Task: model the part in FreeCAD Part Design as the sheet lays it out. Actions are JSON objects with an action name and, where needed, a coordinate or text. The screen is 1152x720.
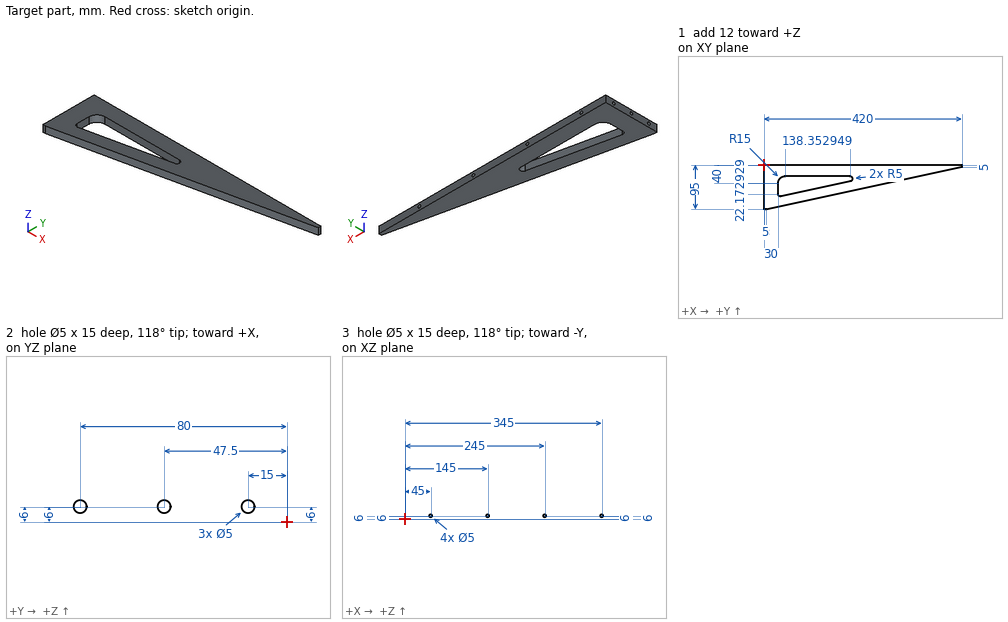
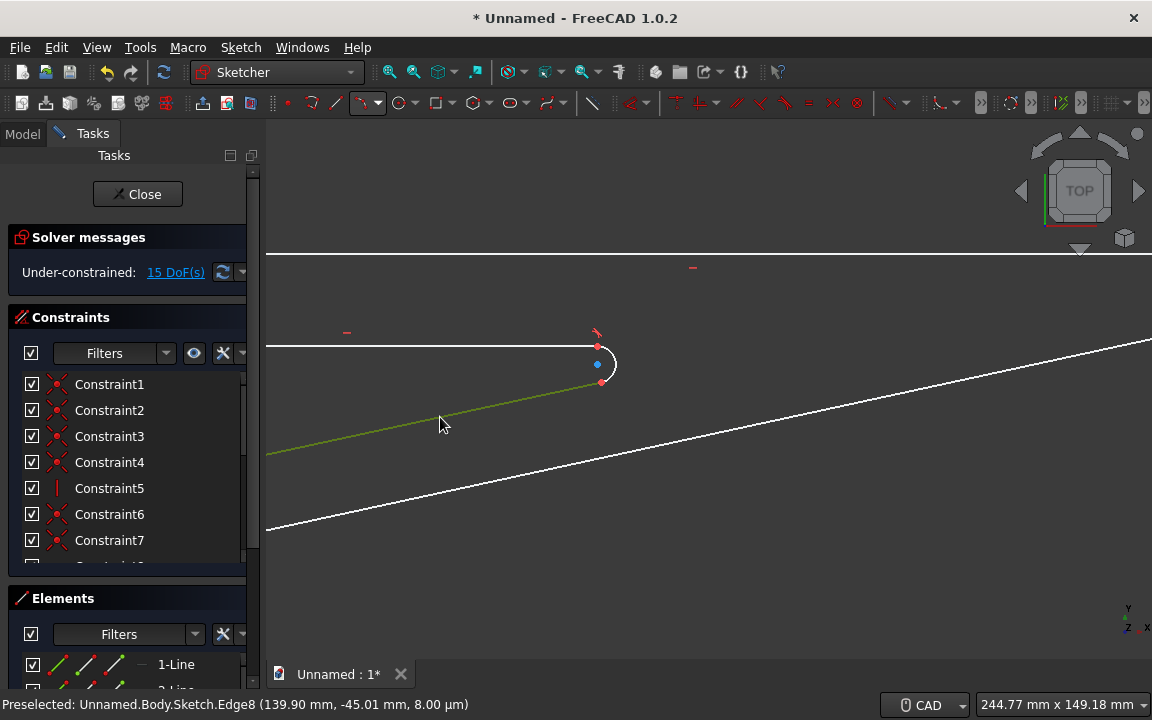
{"action": "left_click", "coordinate": [614, 373]}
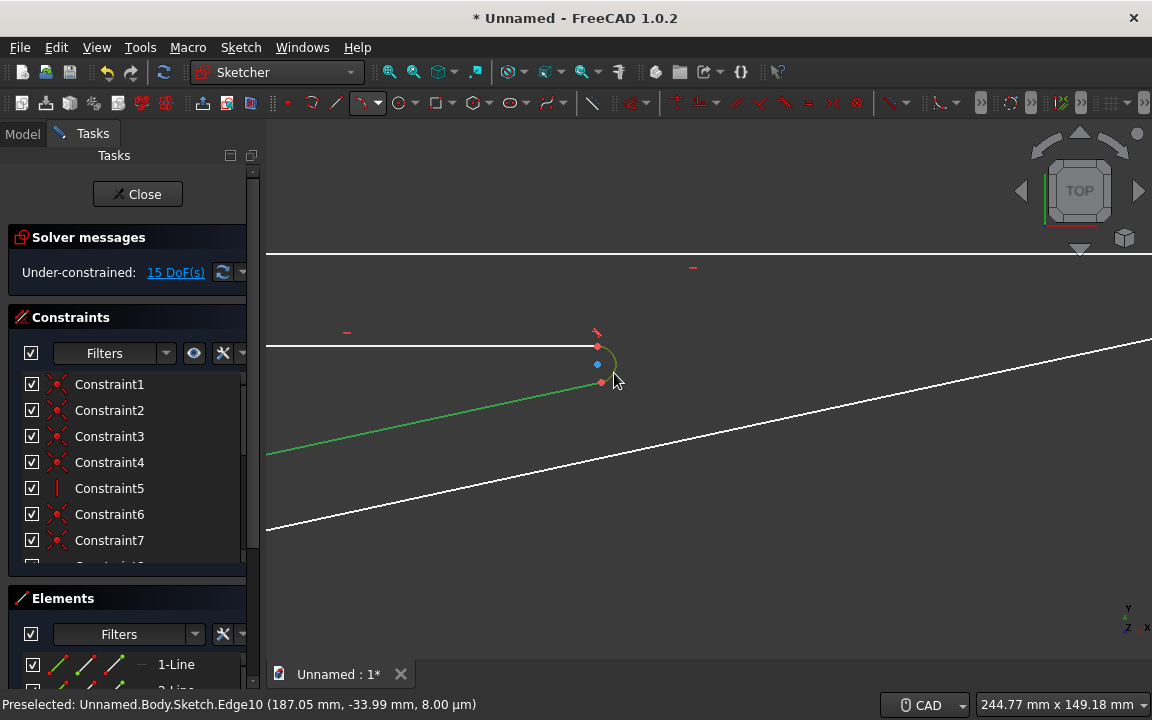
{"action": "left_click", "coordinate": [786, 104]}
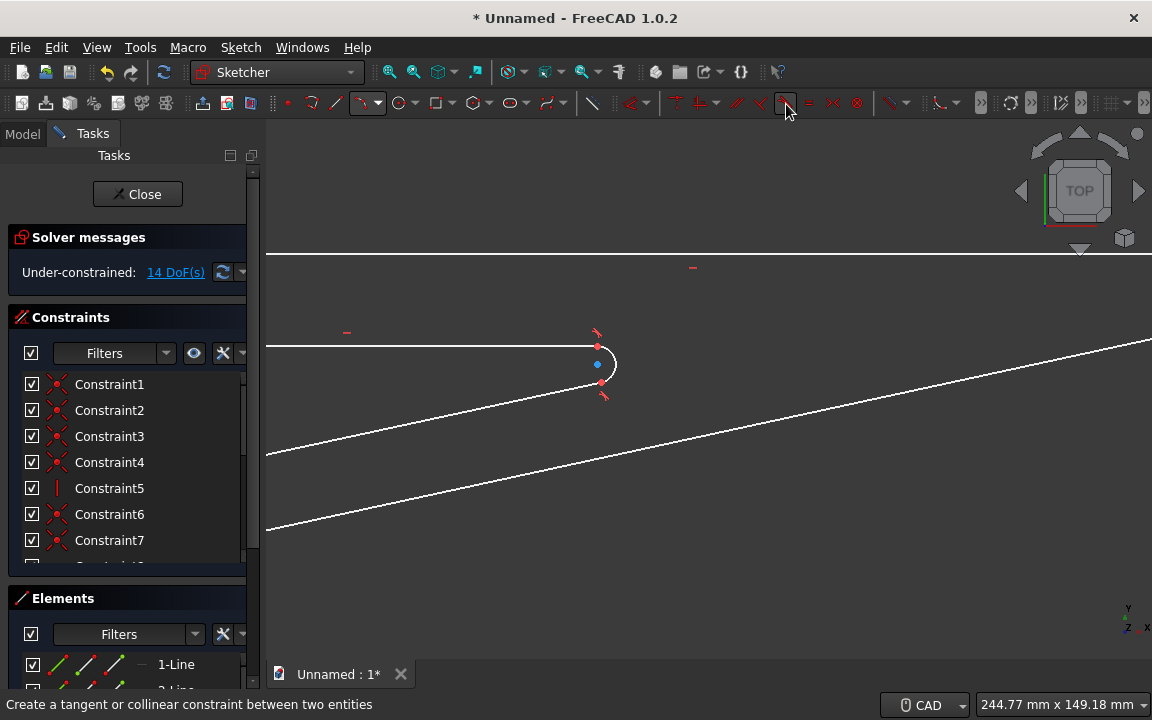
{"action": "left_click", "coordinate": [440, 417]}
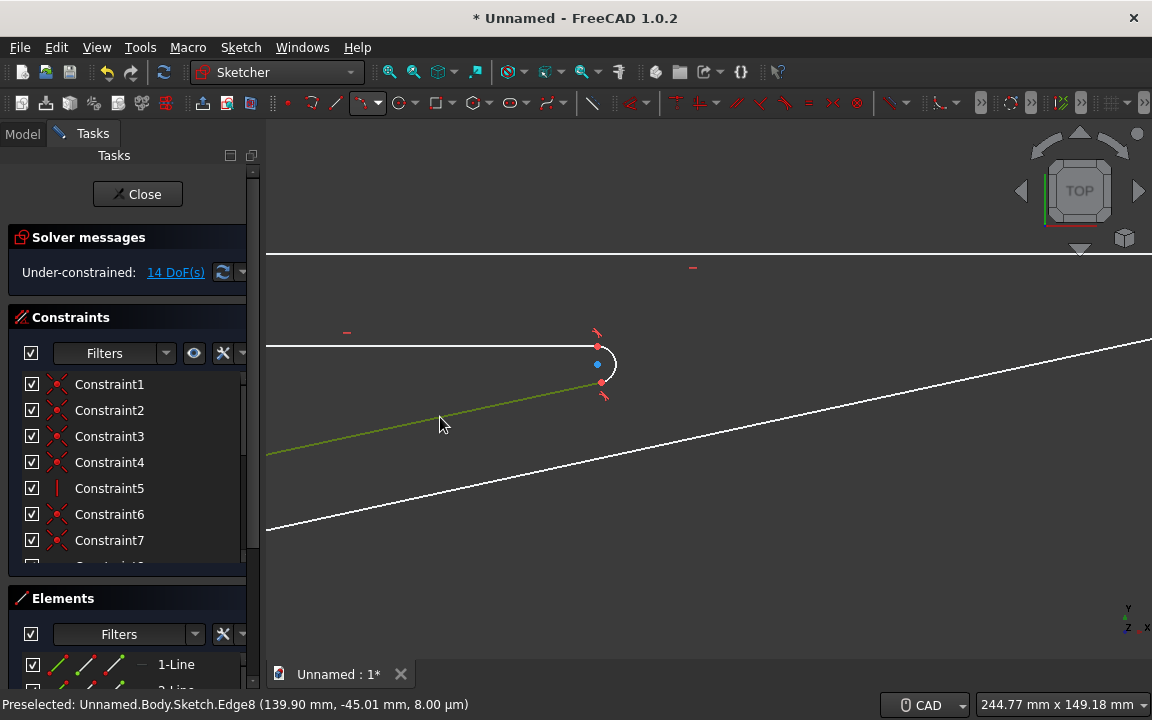
{"action": "scroll", "coordinate": [618, 373], "scroll_direction": "down", "scroll_amount": 6}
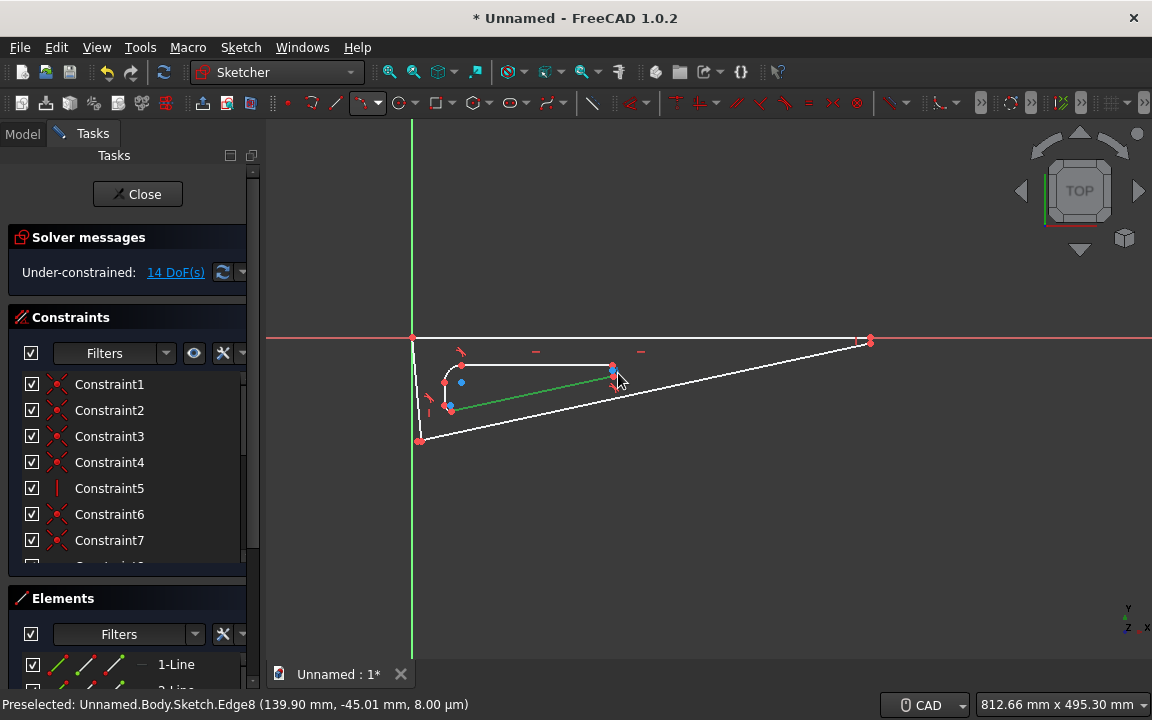
{"action": "scroll", "coordinate": [445, 408], "scroll_direction": "up", "scroll_amount": 8}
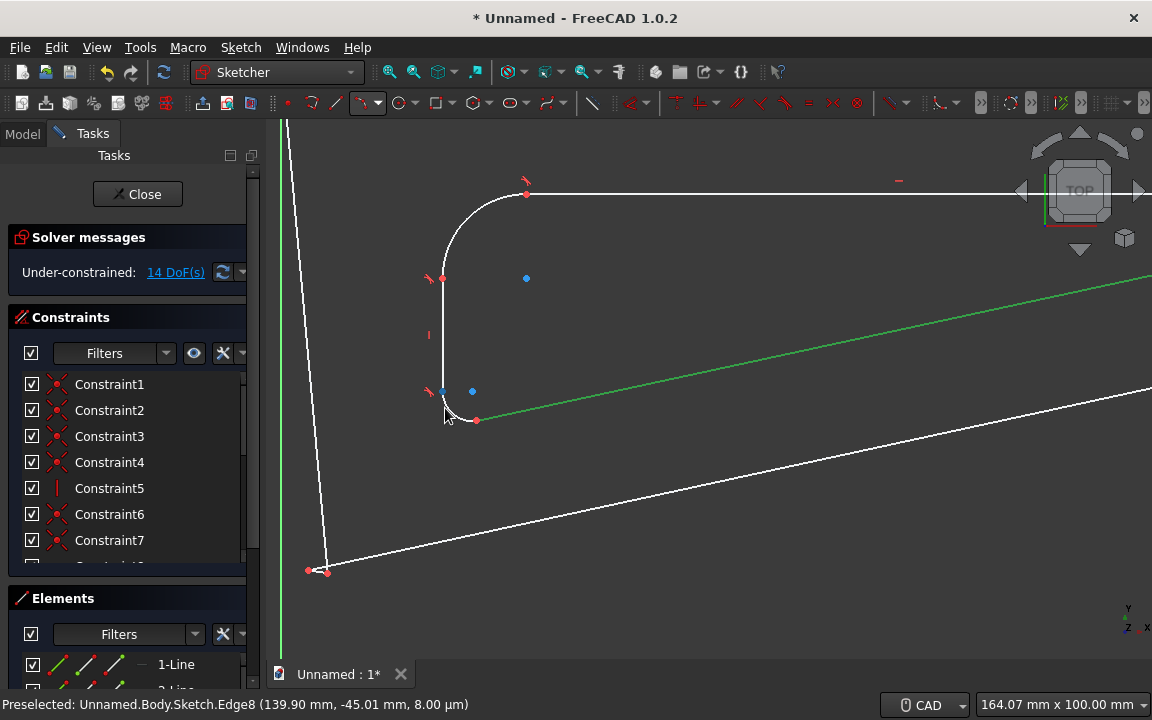
{"action": "left_click", "coordinate": [447, 406]}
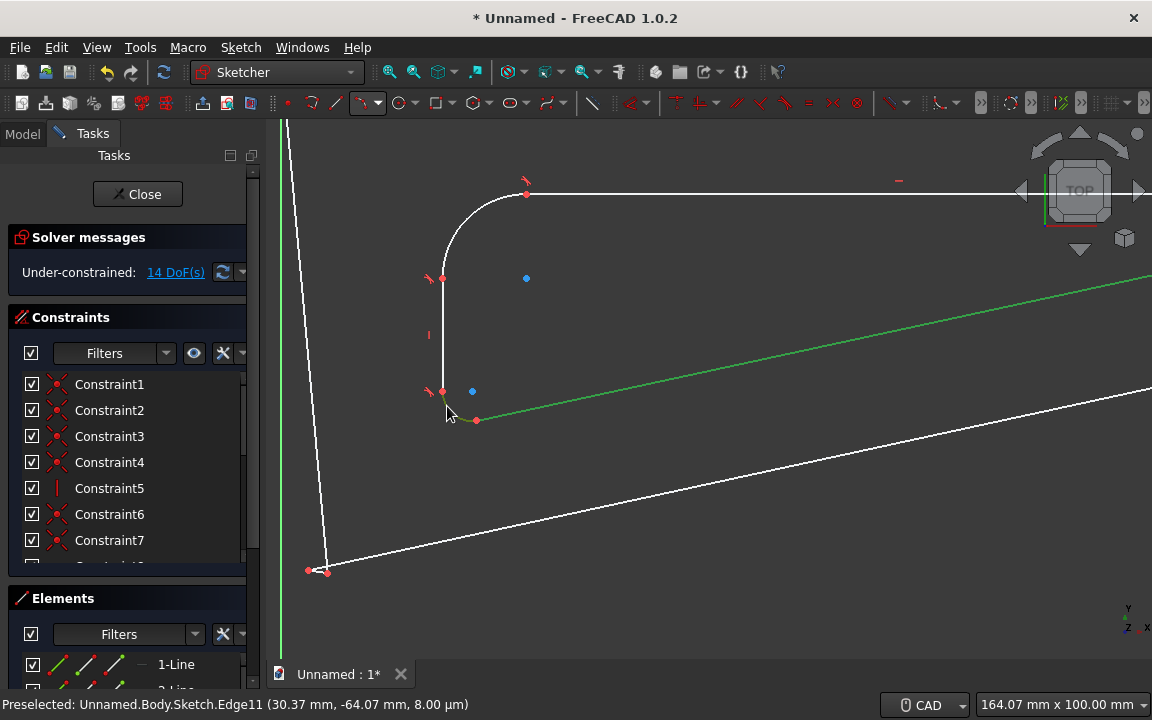
{"action": "left_click", "coordinate": [786, 104]}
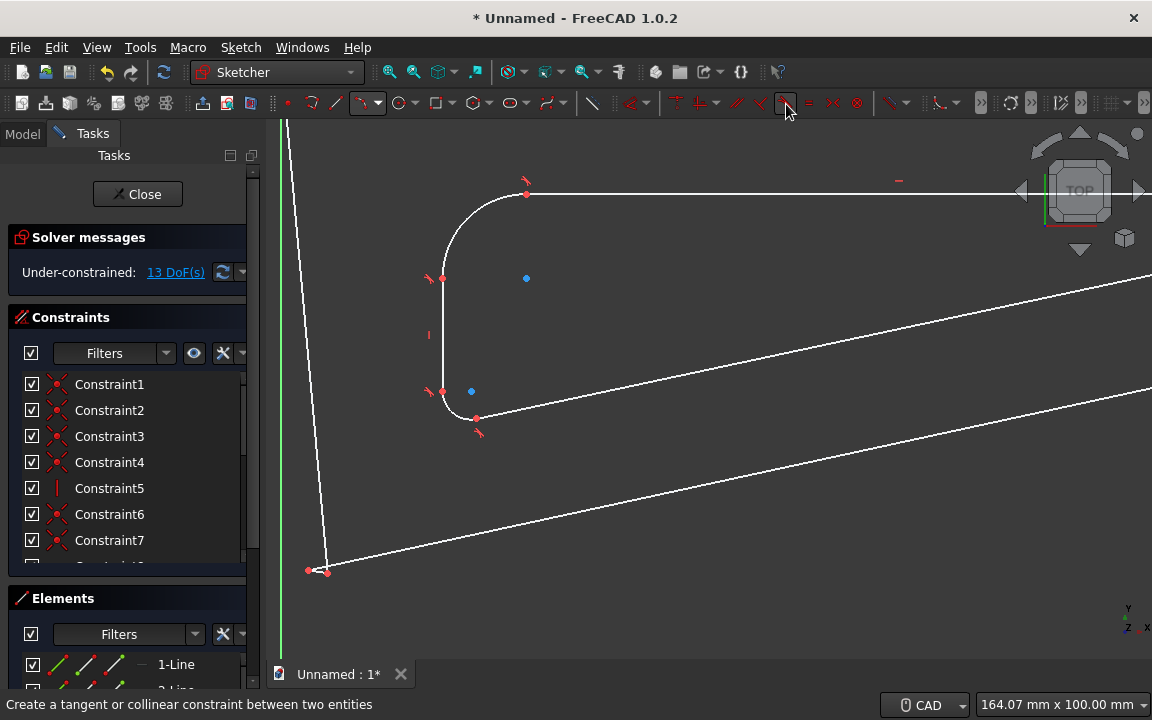
{"action": "left_click", "coordinate": [295, 212]}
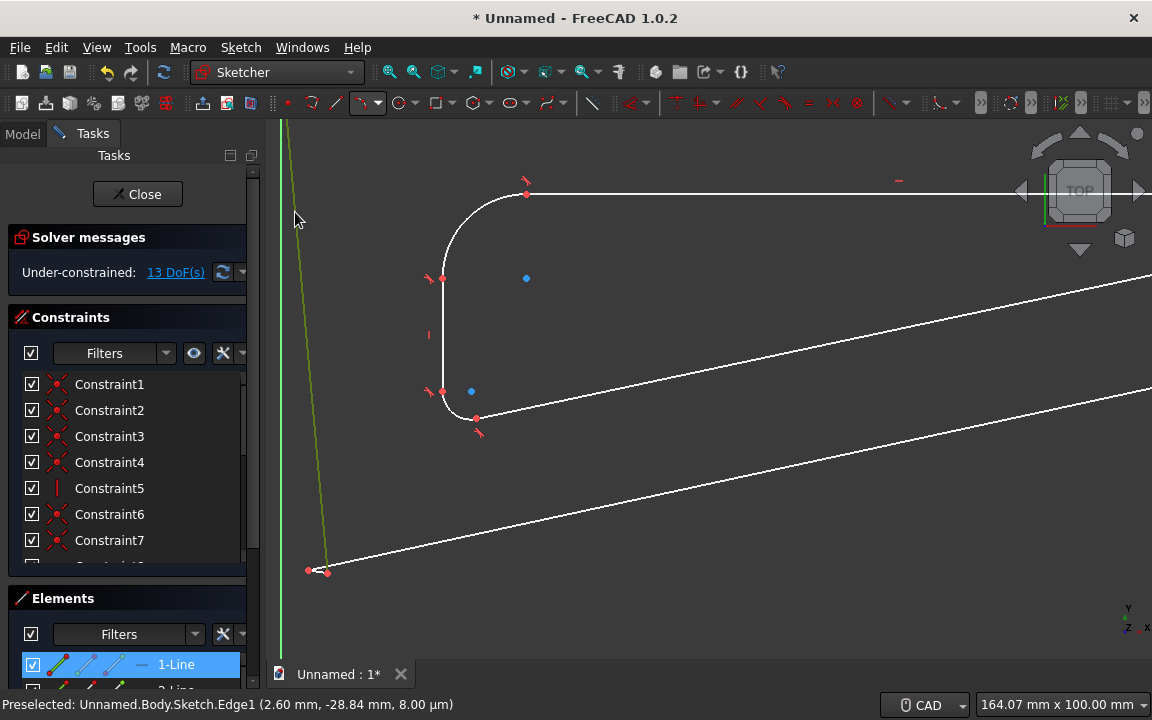
{"action": "key", "text": "v"}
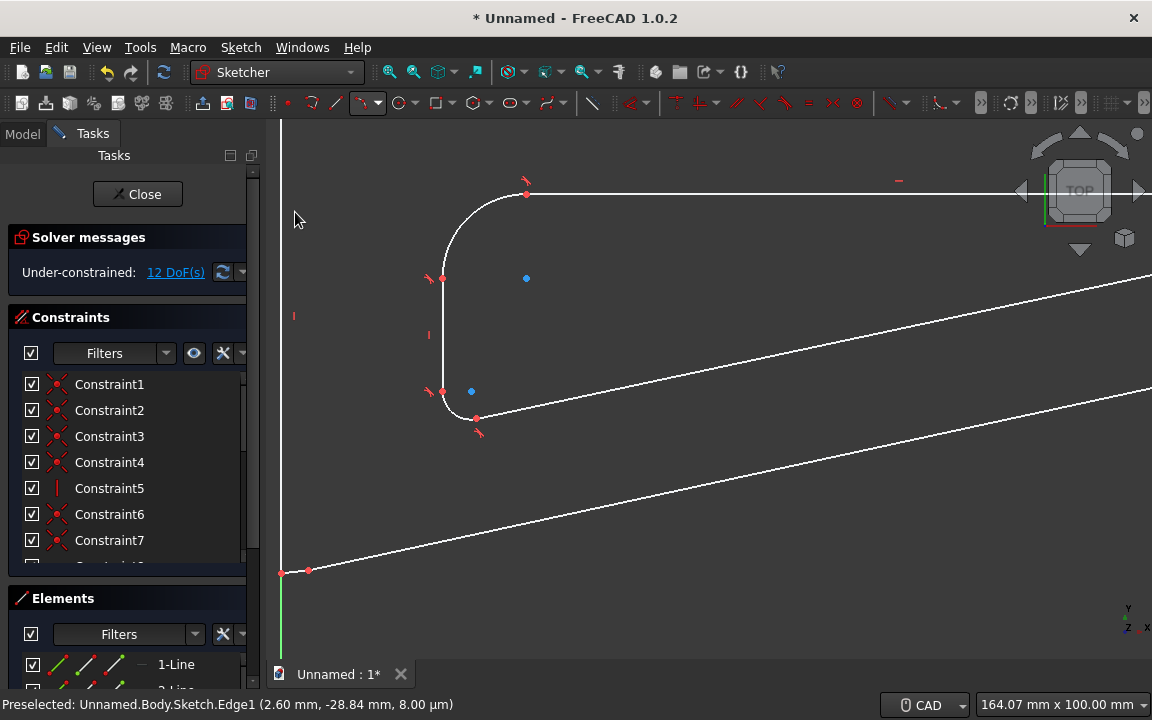
{"action": "scroll", "coordinate": [298, 572], "scroll_direction": "up", "scroll_amount": 2}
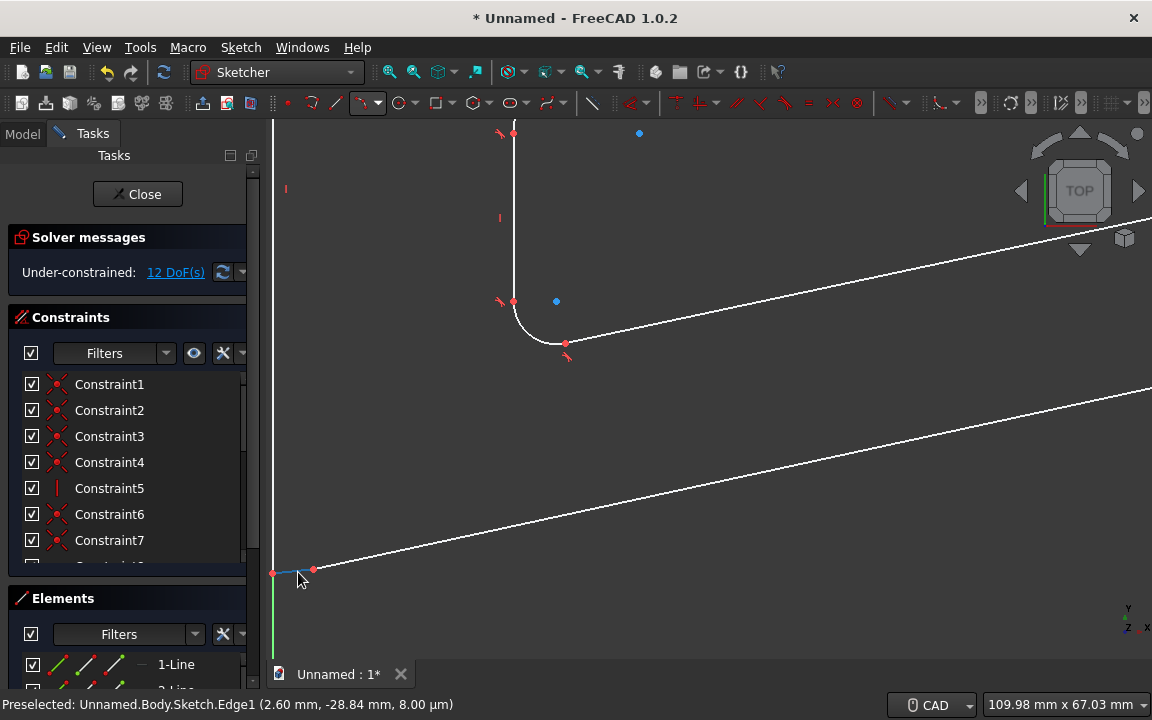
{"action": "left_click", "coordinate": [297, 571]}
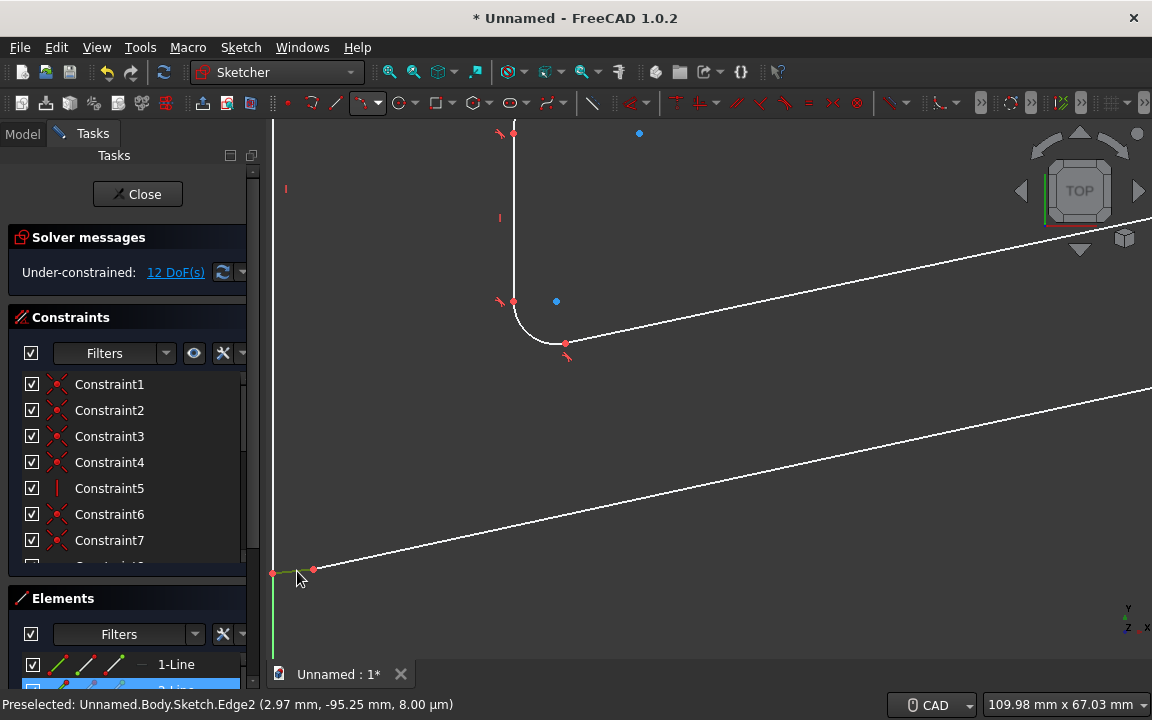
{"action": "left_click", "coordinate": [718, 104]}